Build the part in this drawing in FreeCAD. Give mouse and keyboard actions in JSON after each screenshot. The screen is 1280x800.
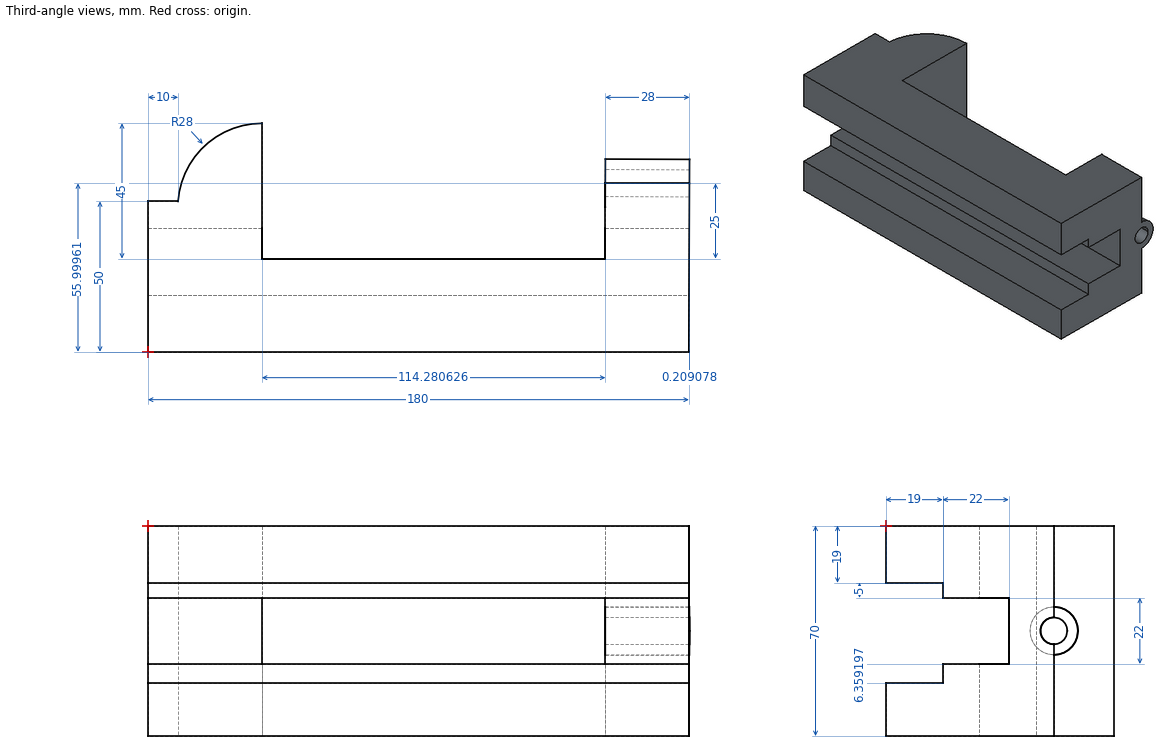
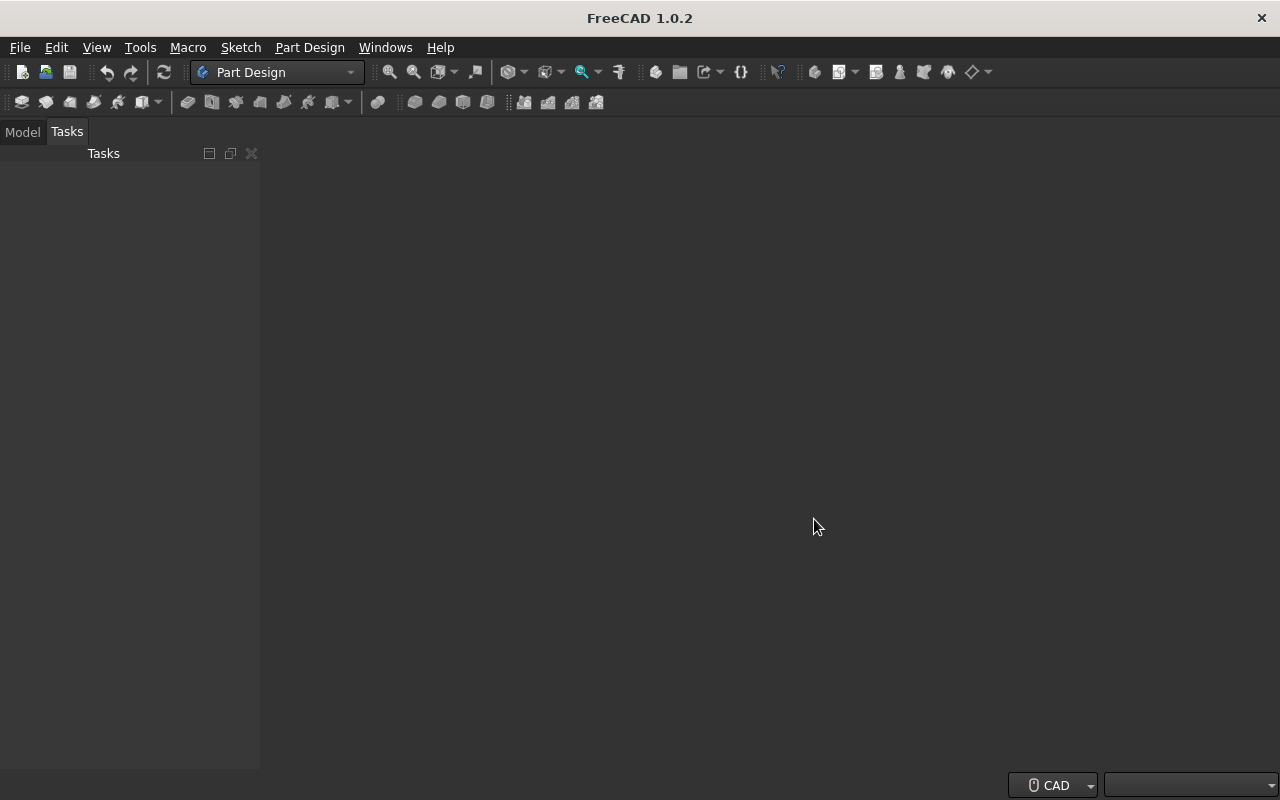
{"action": "left_click", "coordinate": [22, 72]}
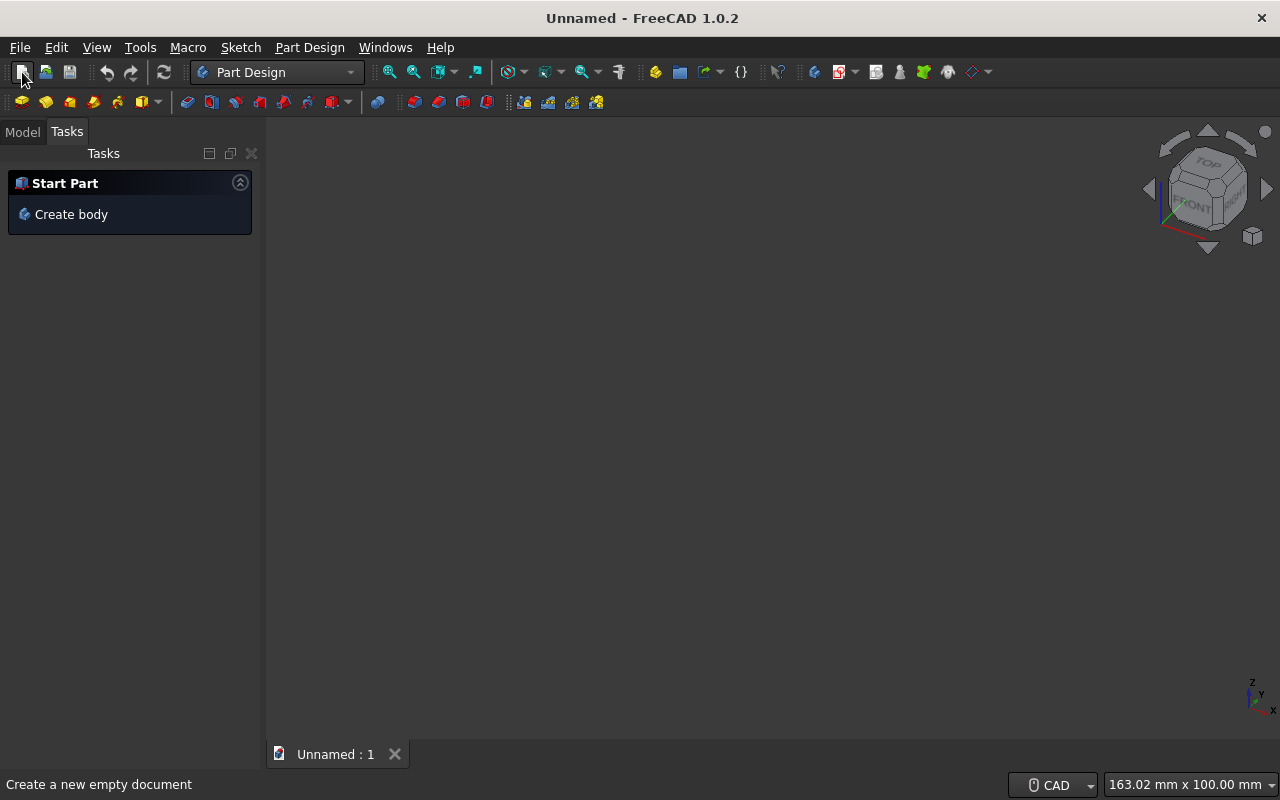
{"action": "left_click", "coordinate": [840, 72]}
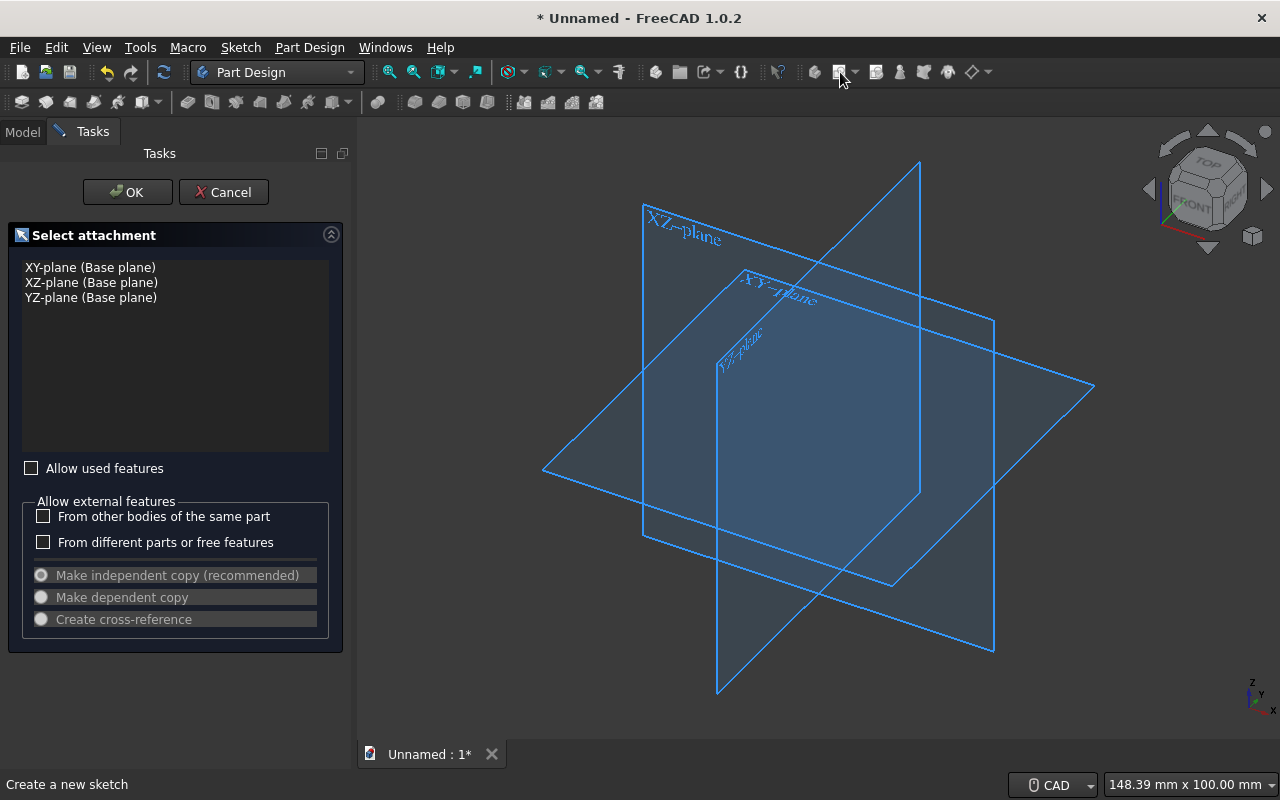
{"action": "left_click", "coordinate": [82, 268]}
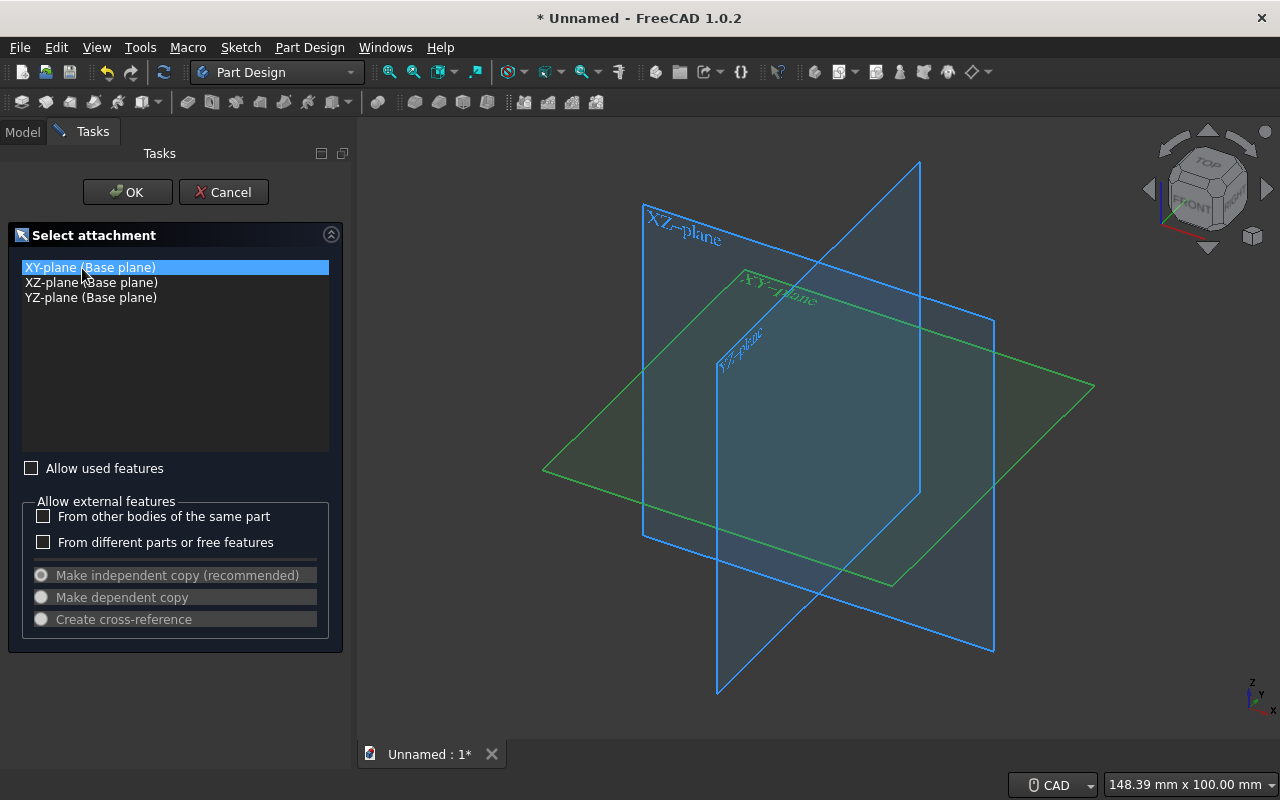
{"action": "left_click", "coordinate": [128, 192]}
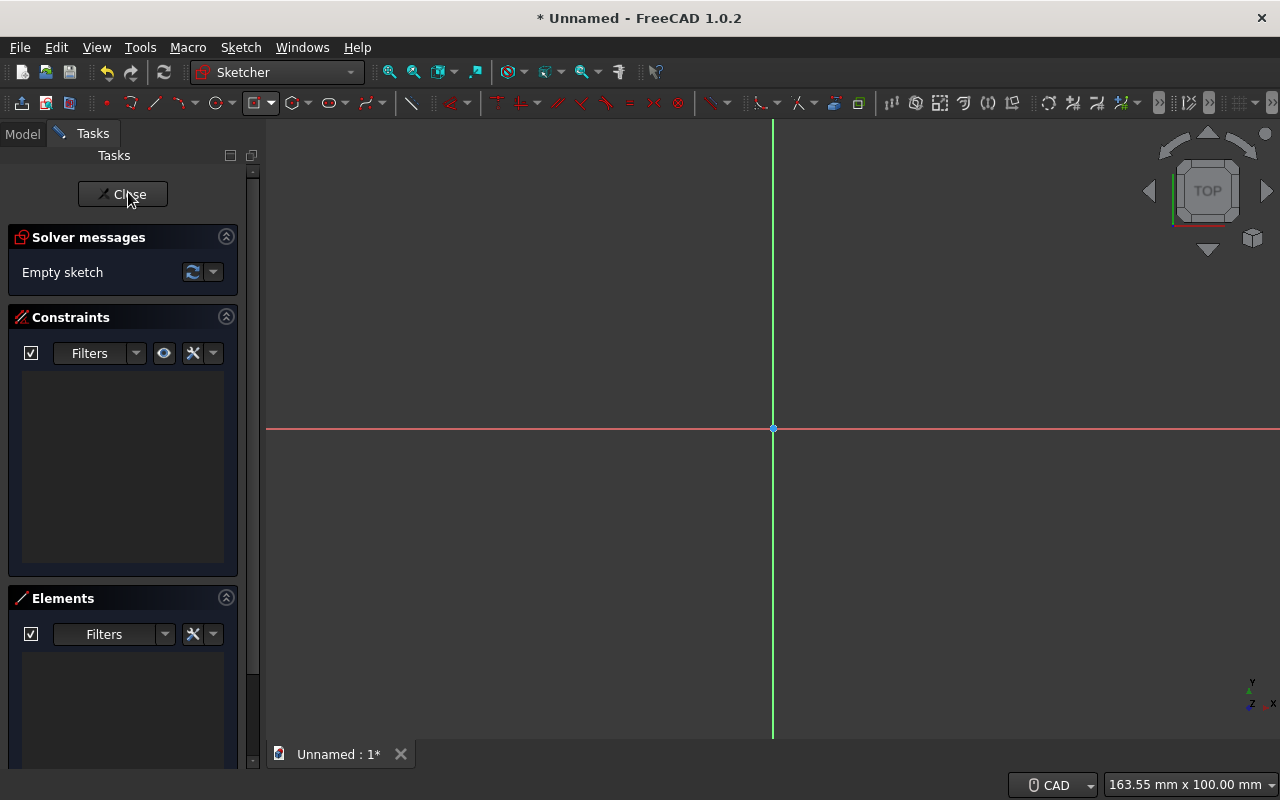
{"action": "scroll", "coordinate": [294, 621], "scroll_direction": "down", "scroll_amount": 4}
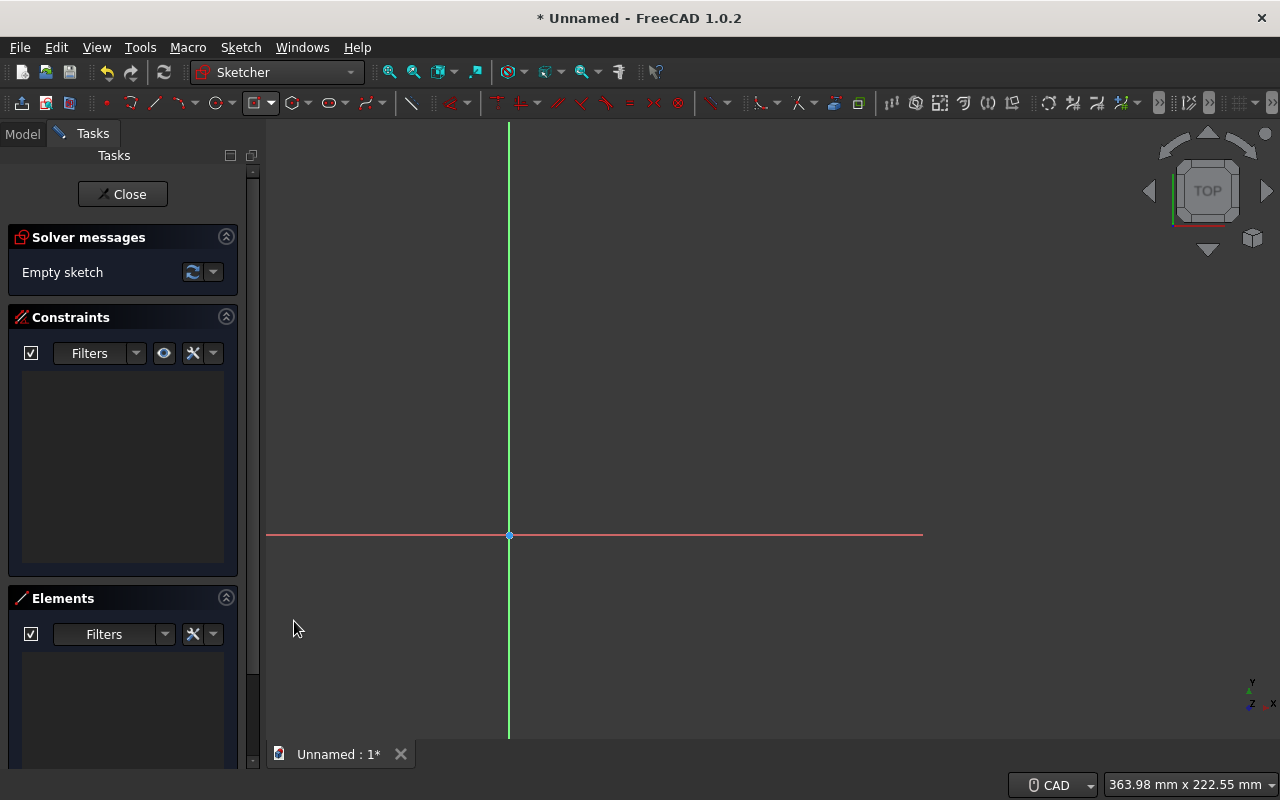
{"action": "left_click", "coordinate": [132, 104]}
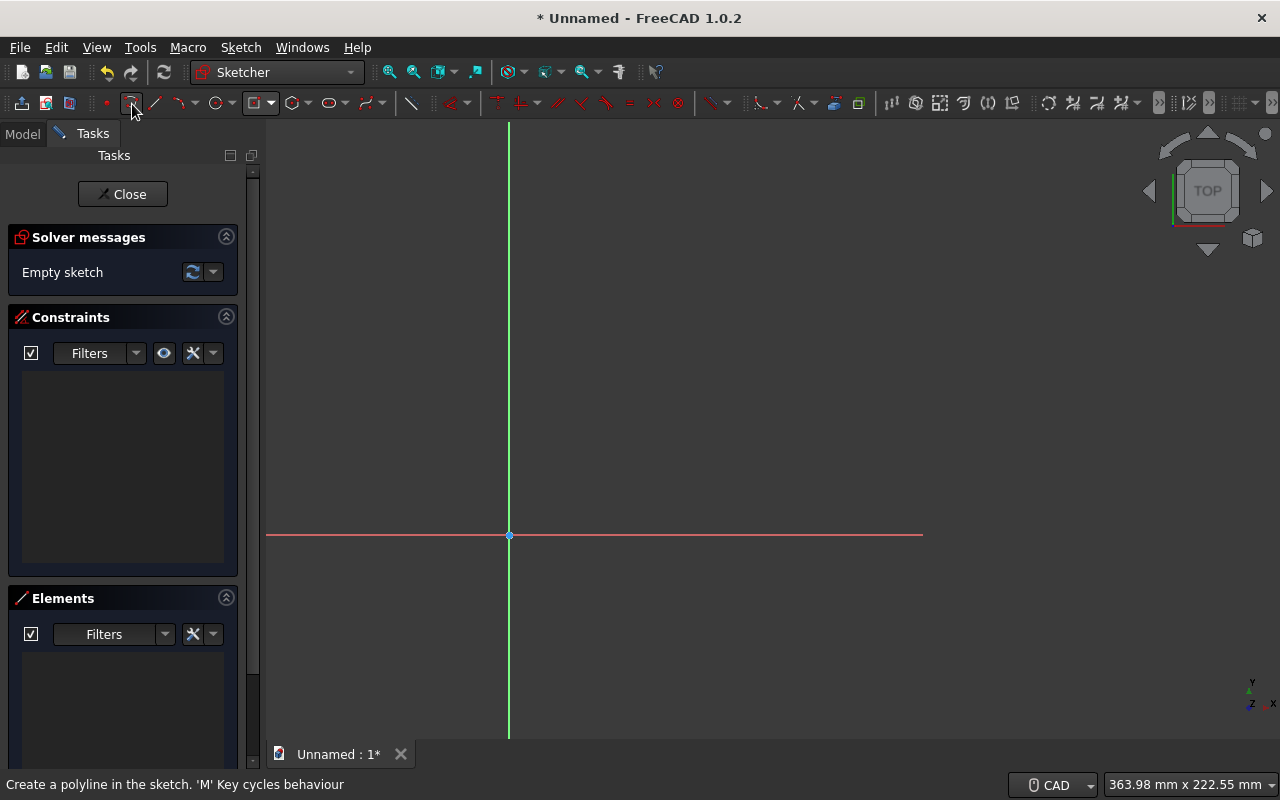
{"action": "left_click", "coordinate": [537, 396]}
{"action": "left_click", "coordinate": [509, 396]}
{"action": "left_click", "coordinate": [509, 535]}
{"action": "left_click", "coordinate": [1011, 526]}
{"action": "left_click", "coordinate": [1020, 379]}
{"action": "left_click", "coordinate": [933, 379]}
{"action": "left_click", "coordinate": [933, 449]}
{"action": "left_click", "coordinate": [615, 449]}
{"action": "left_click", "coordinate": [615, 323]}
{"action": "right_click", "coordinate": [615, 323]}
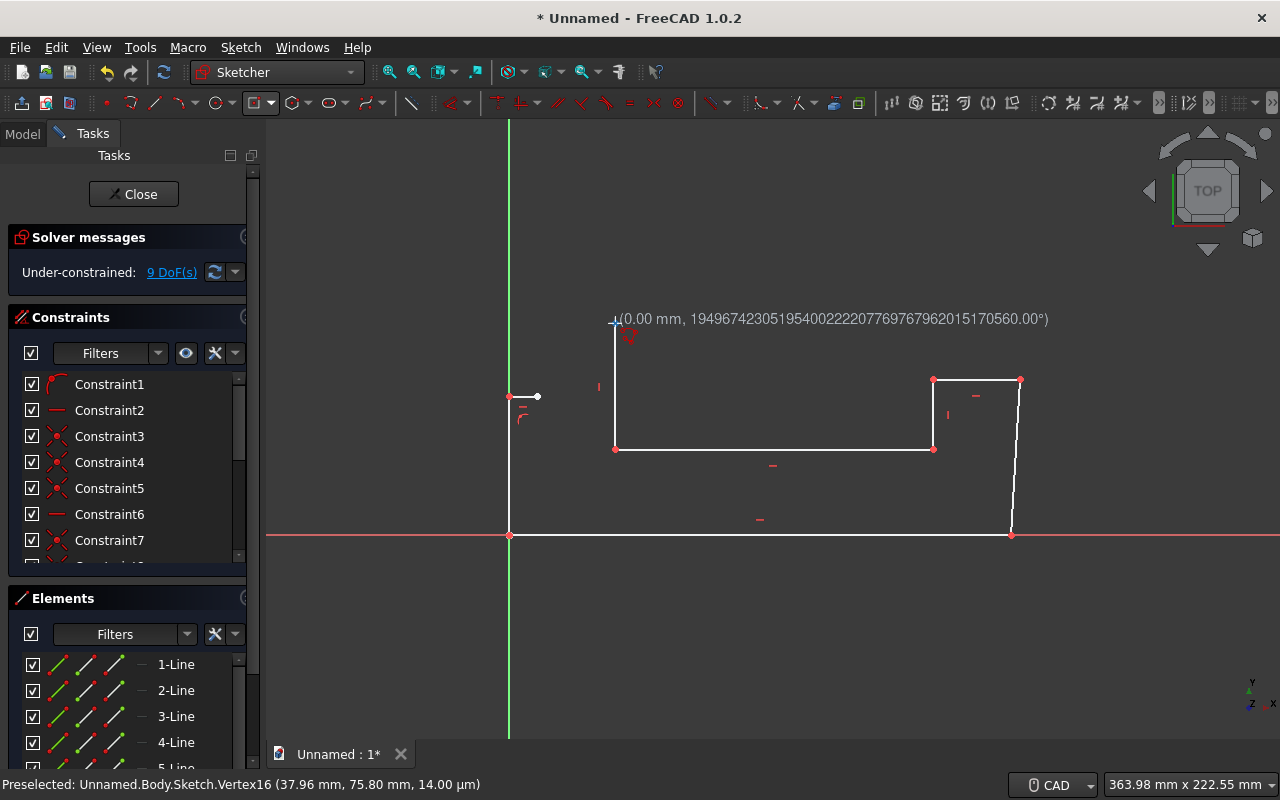
{"action": "left_click", "coordinate": [180, 104]}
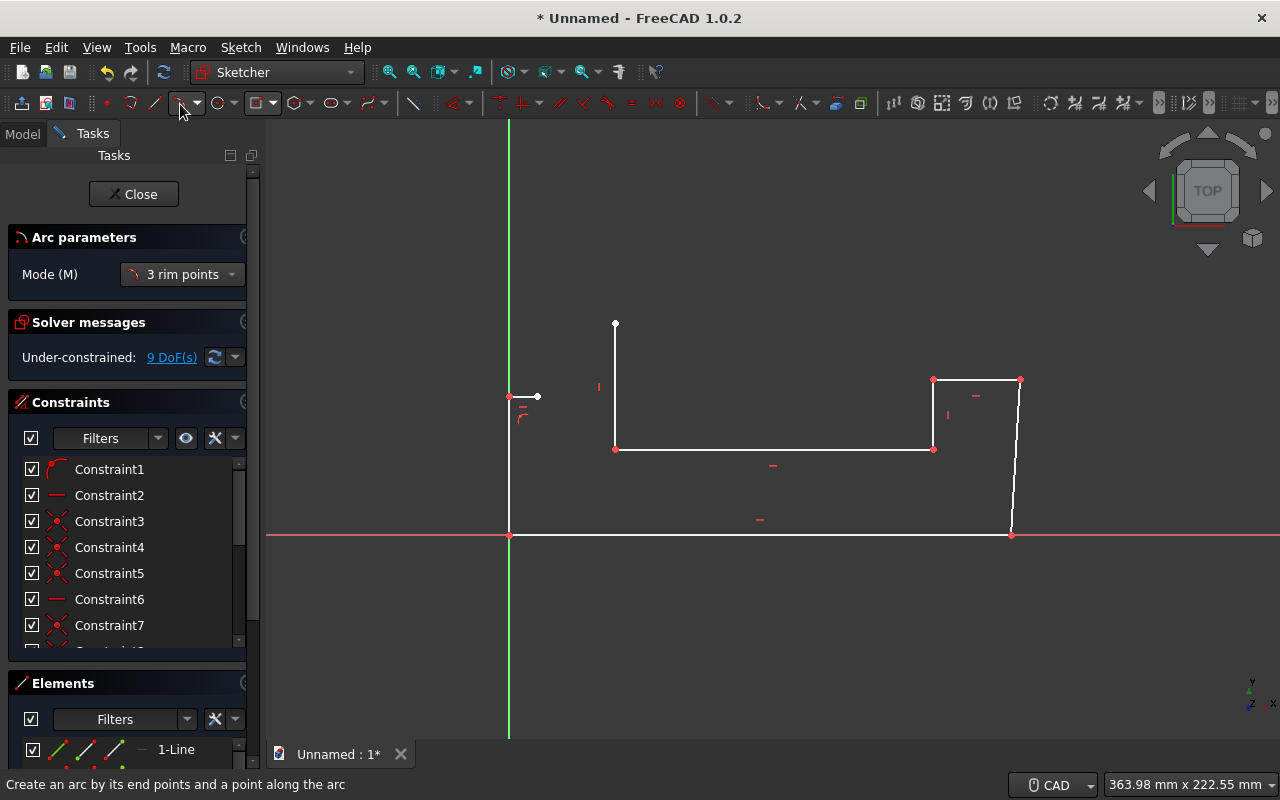
{"action": "left_click", "coordinate": [615, 324]}
{"action": "left_click", "coordinate": [537, 397]}
{"action": "left_click", "coordinate": [562, 344]}
{"action": "key", "text": "Escape"}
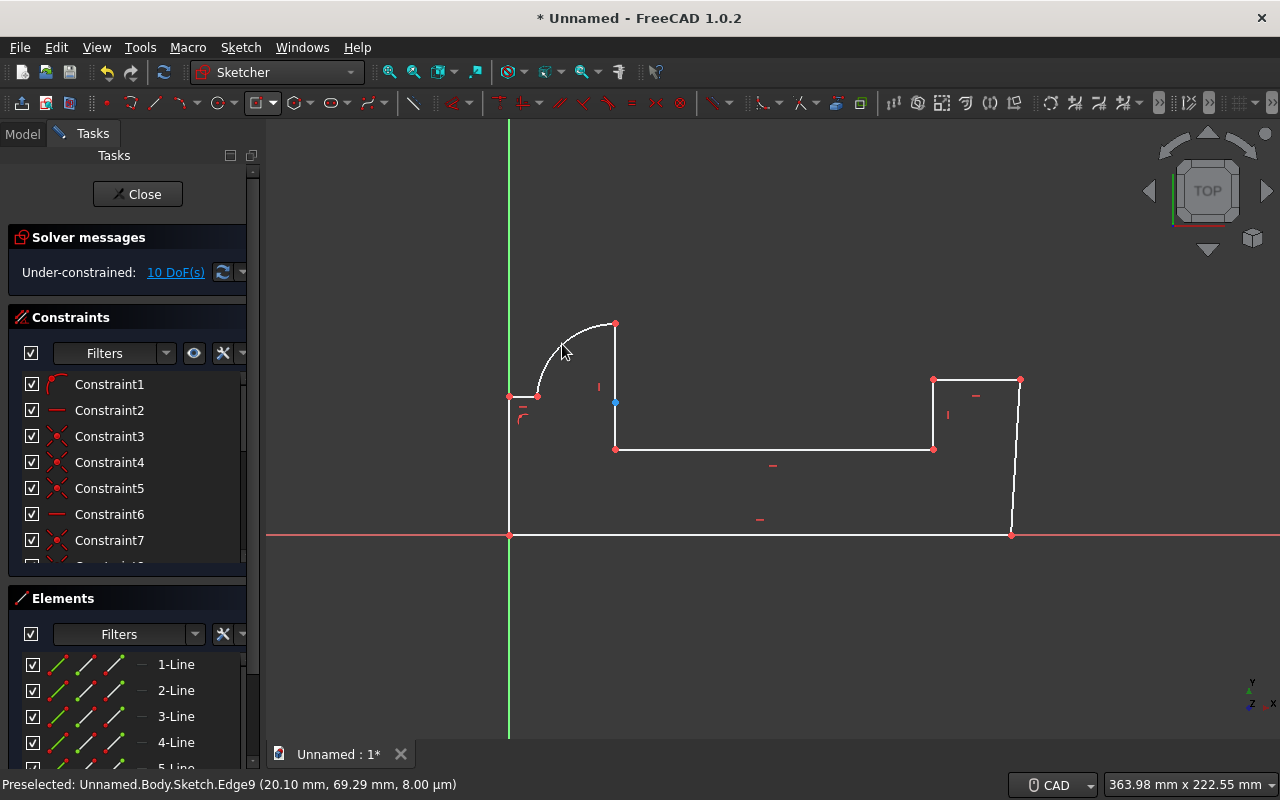
{"action": "left_click", "coordinate": [452, 104]}